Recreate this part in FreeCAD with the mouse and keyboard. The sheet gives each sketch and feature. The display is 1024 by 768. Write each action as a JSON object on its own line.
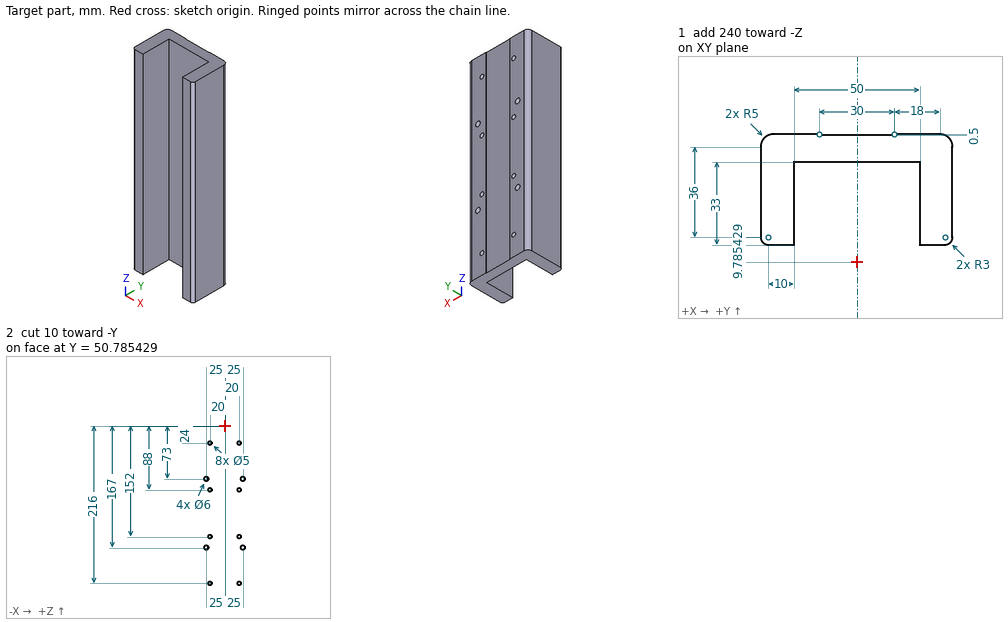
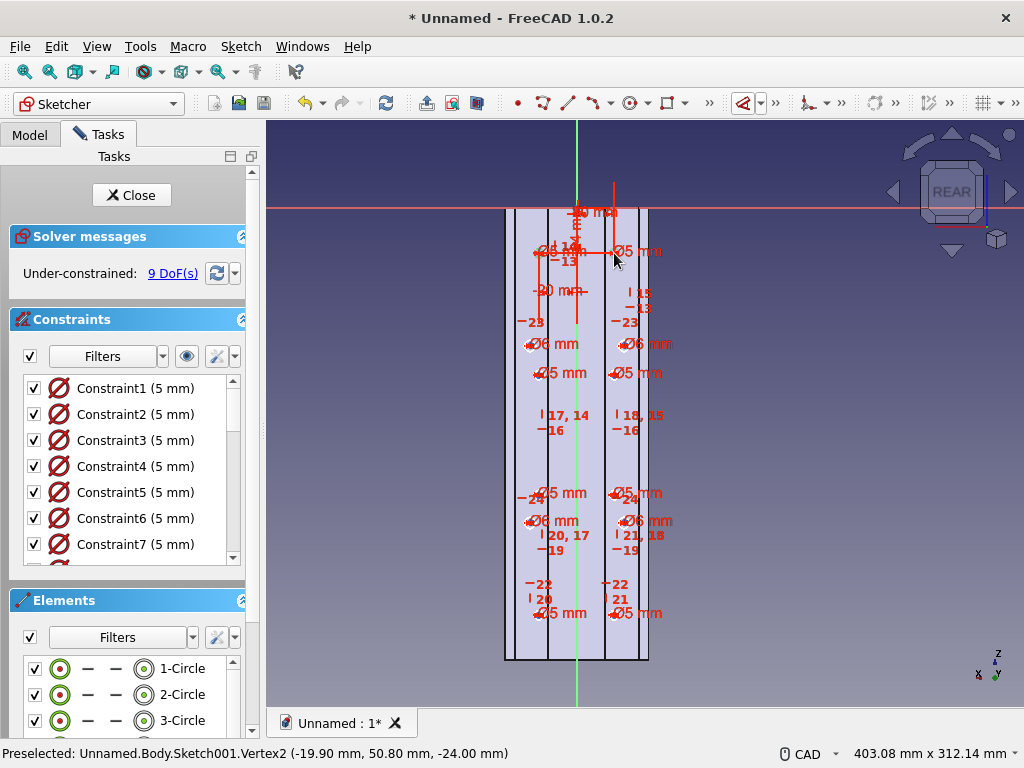
{"action": "left_click", "coordinate": [539, 375]}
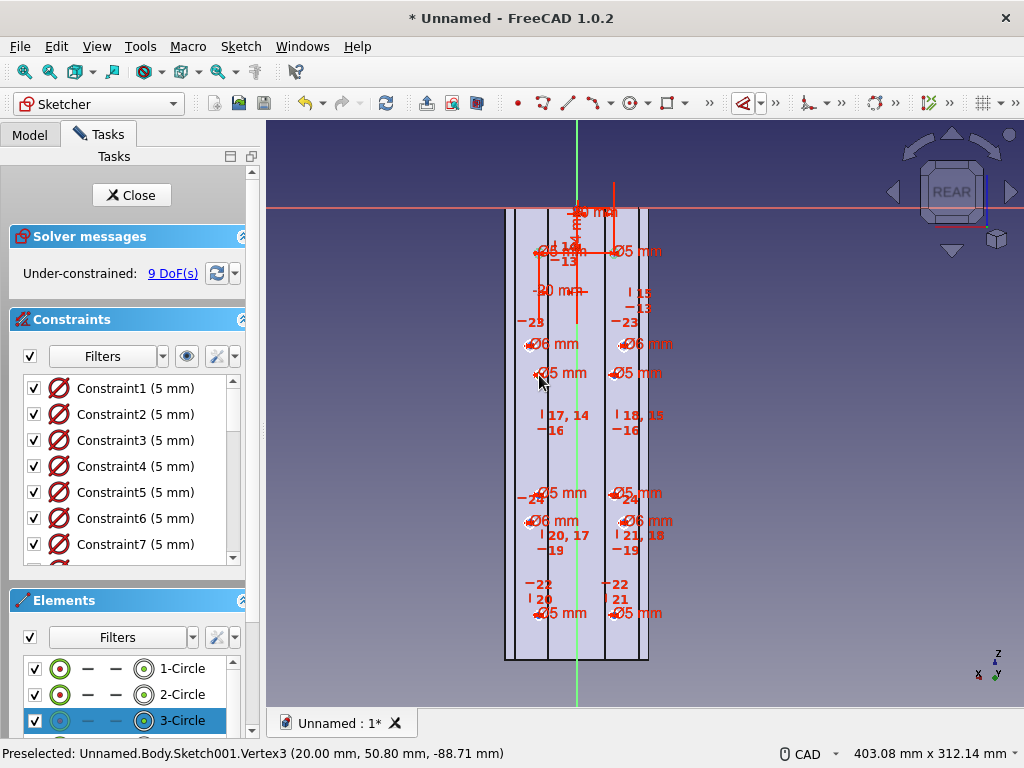
{"action": "left_click", "coordinate": [760, 104]}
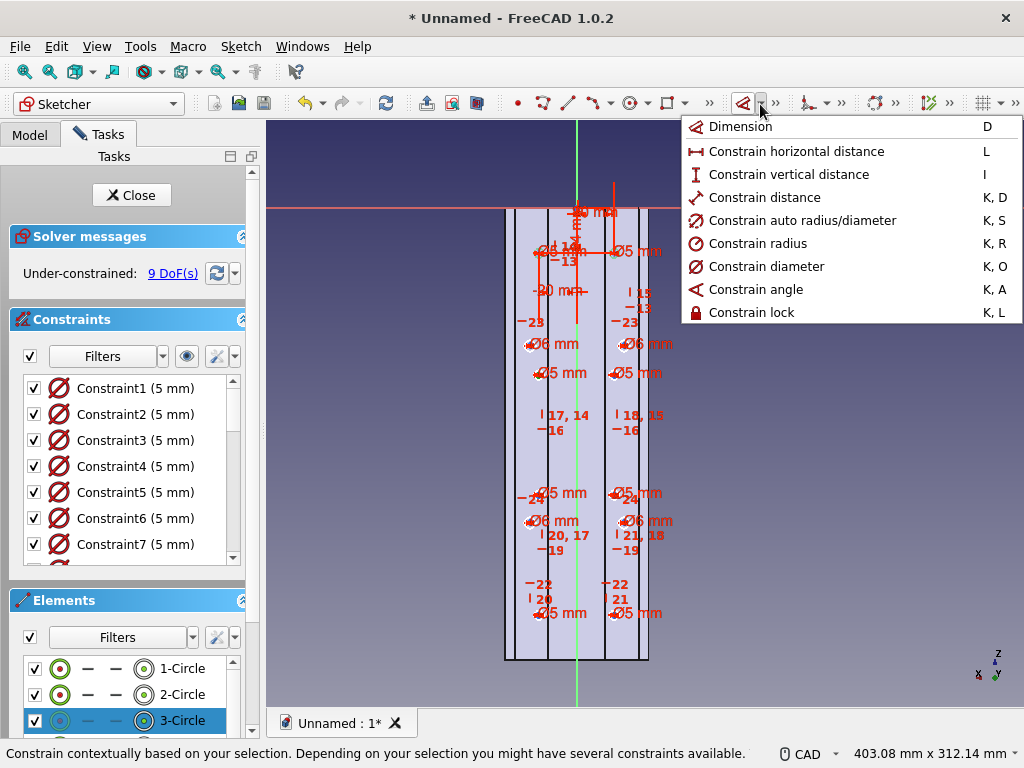
{"action": "left_click", "coordinate": [852, 174]}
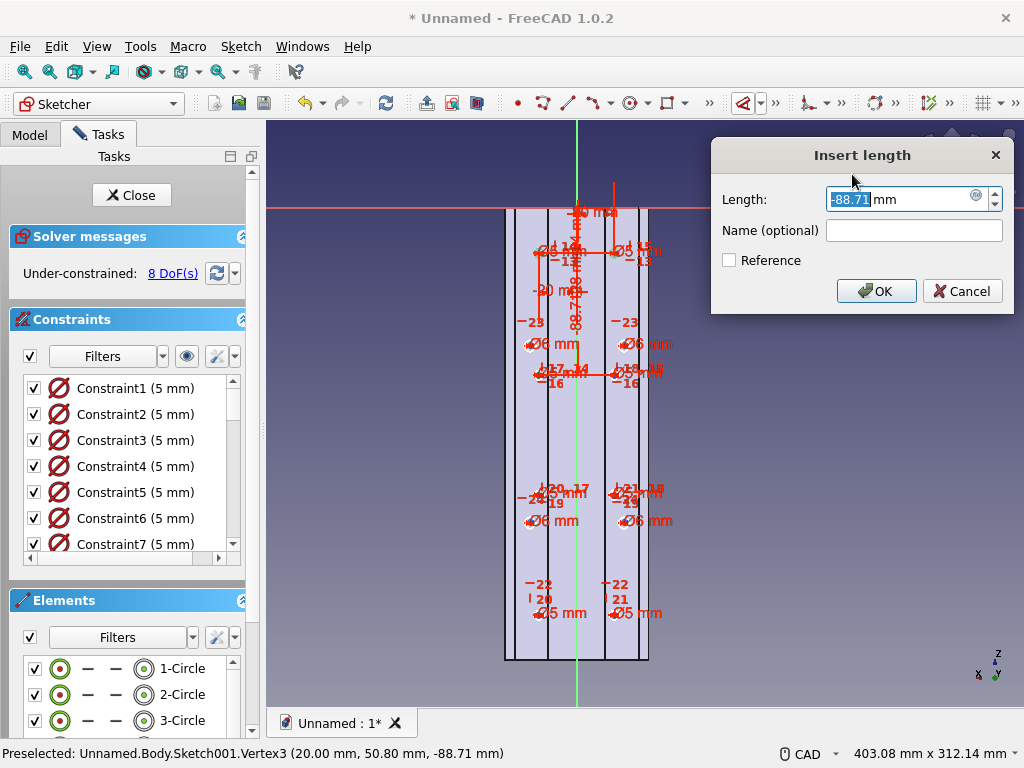
{"action": "type", "text": "-88"}
{"action": "key", "text": "Return"}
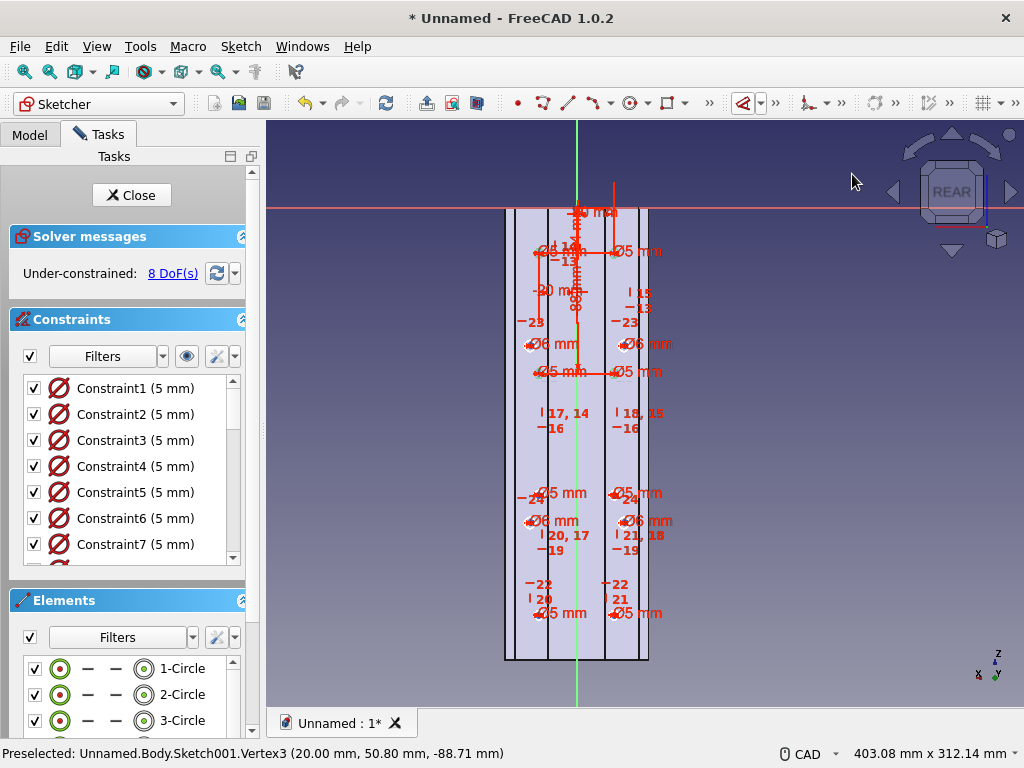
{"action": "left_click", "coordinate": [530, 346]}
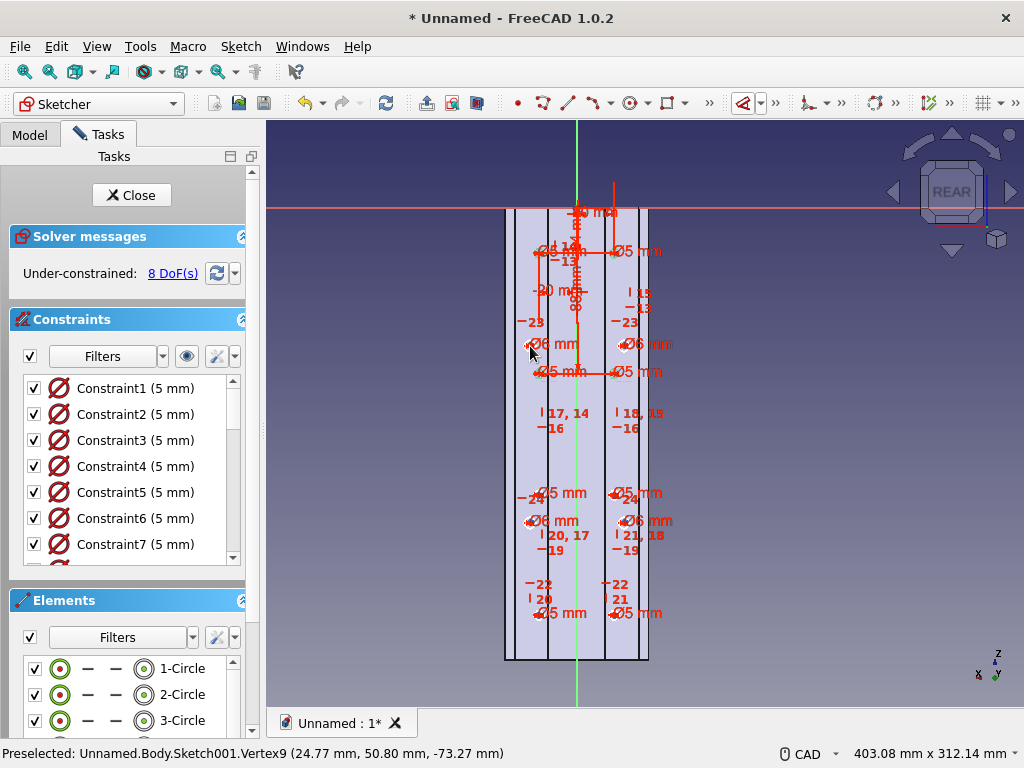
{"action": "left_click", "coordinate": [760, 104]}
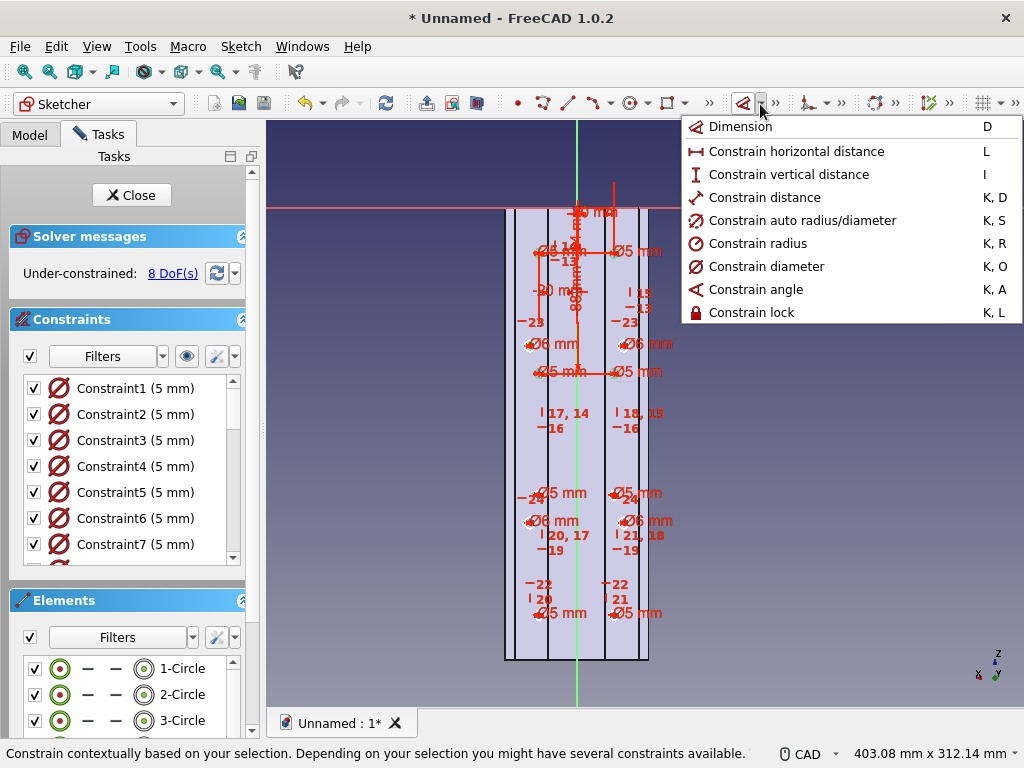
{"action": "left_click", "coordinate": [852, 152]}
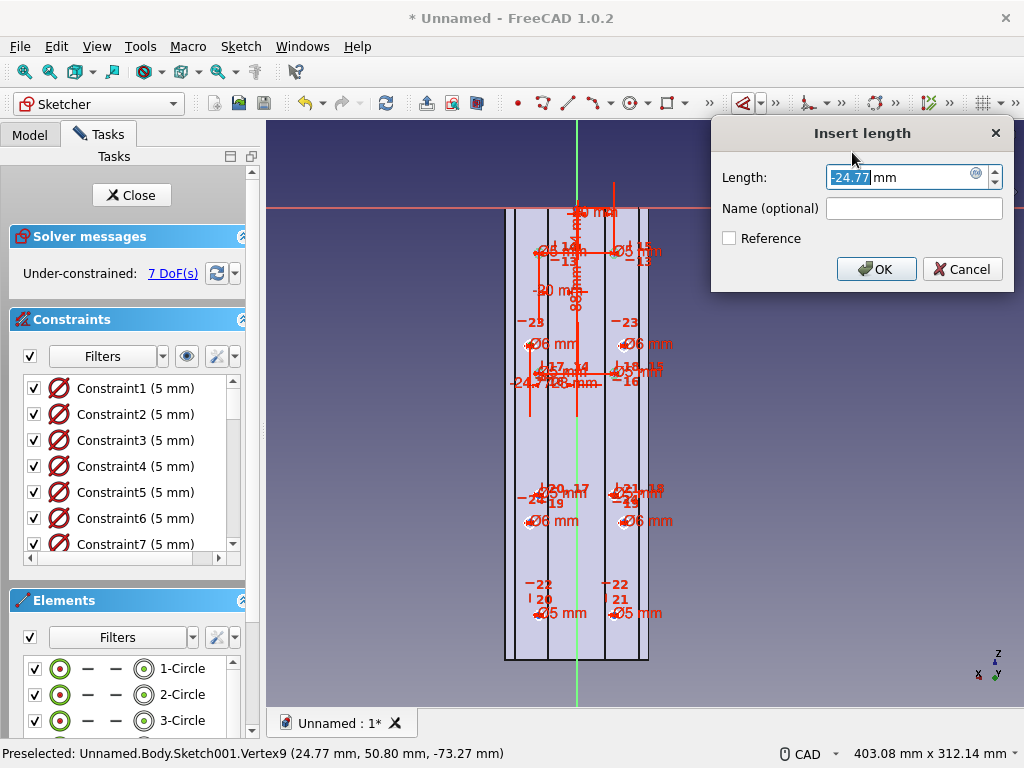
{"action": "type", "text": "-25"}
{"action": "key", "text": "Return"}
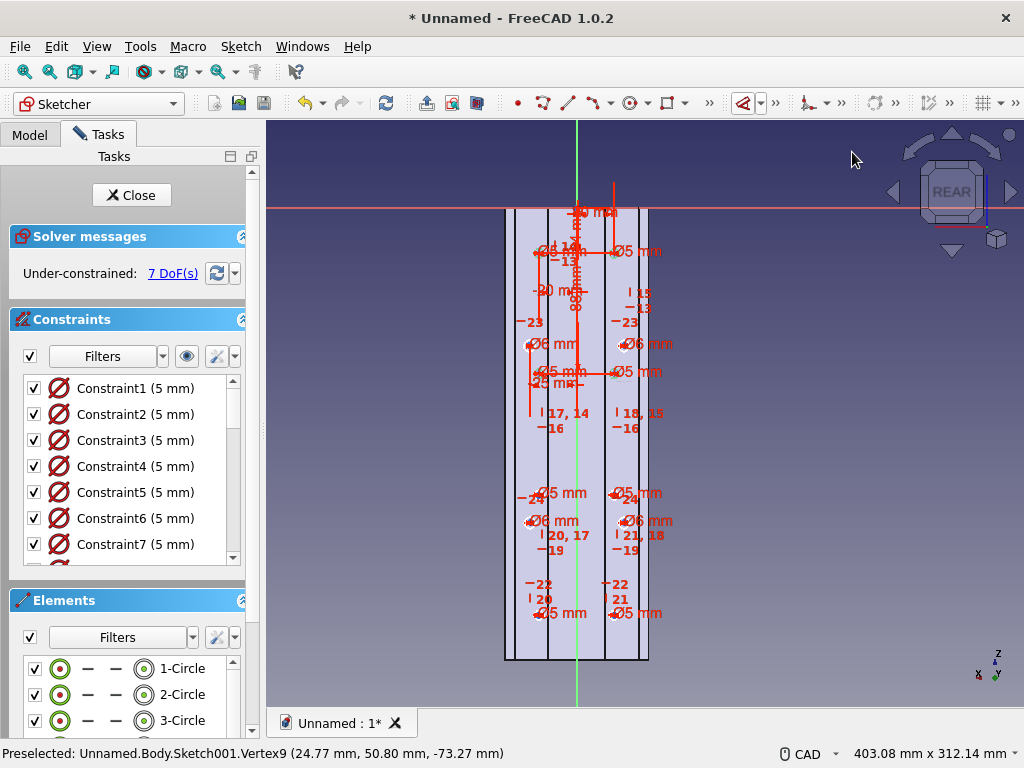
{"action": "left_click", "coordinate": [530, 346]}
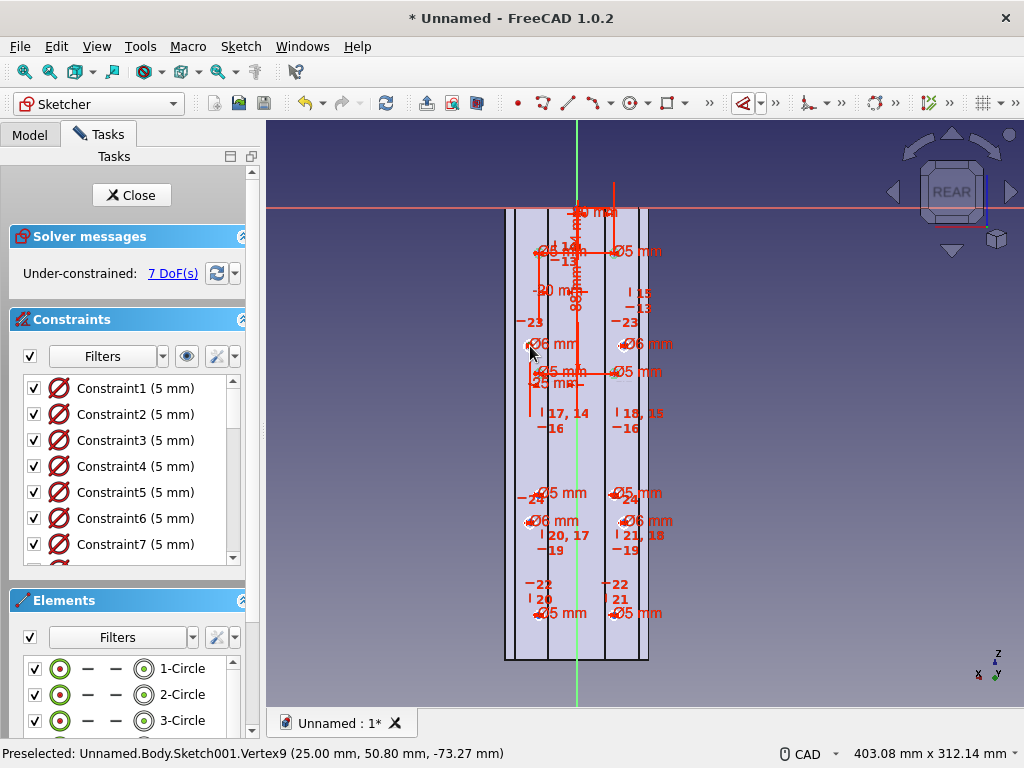
{"action": "left_click", "coordinate": [760, 104]}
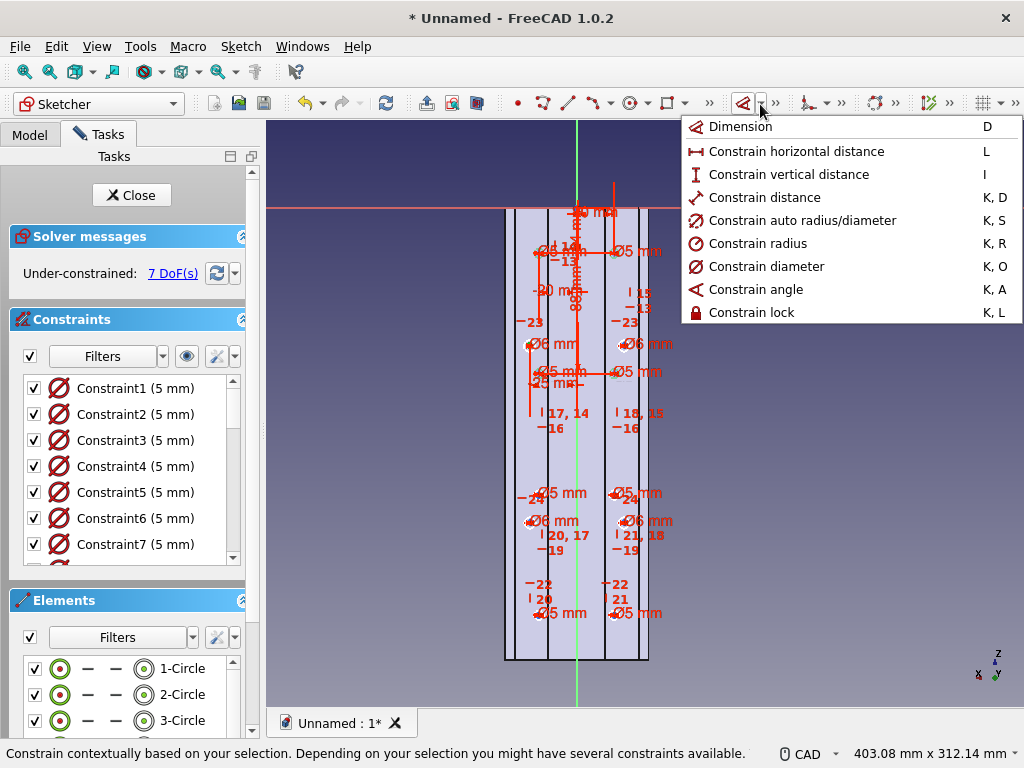
{"action": "left_click", "coordinate": [852, 174]}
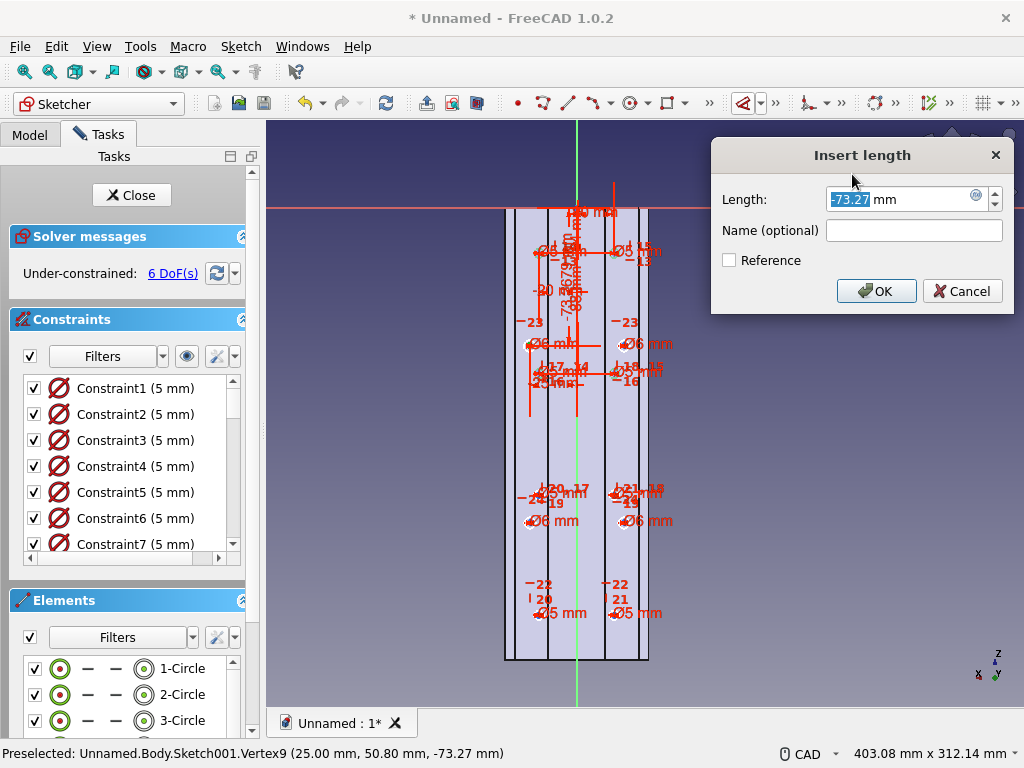
{"action": "type", "text": "-73"}
{"action": "key", "text": "Return"}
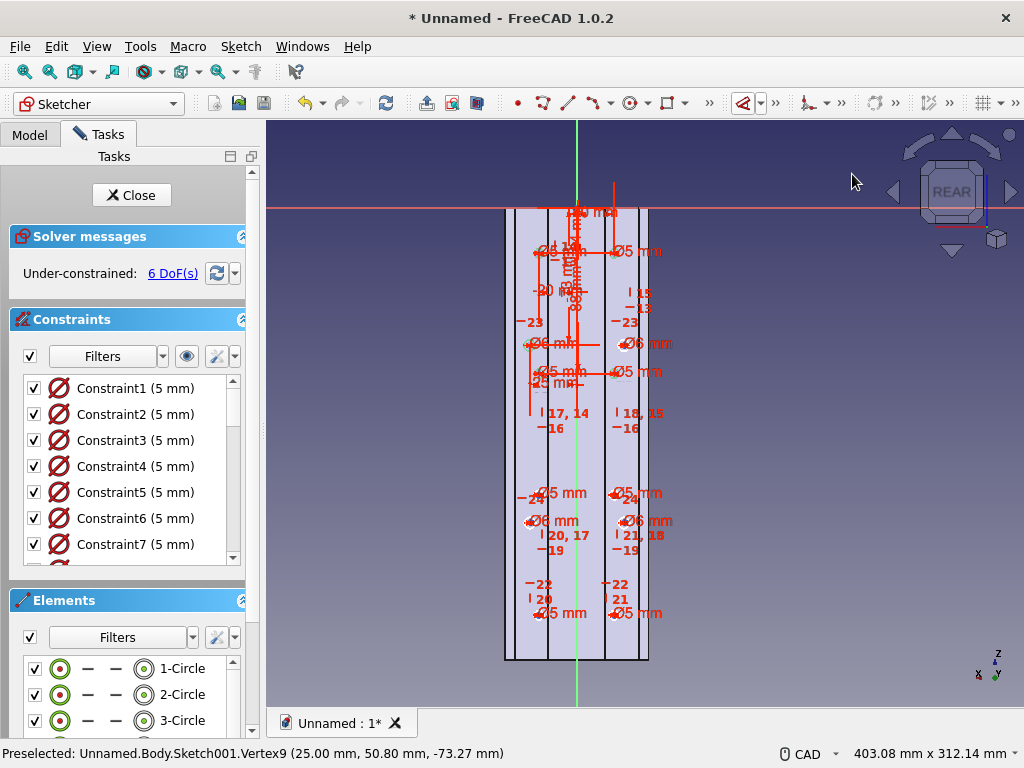
{"action": "left_click", "coordinate": [624, 345]}